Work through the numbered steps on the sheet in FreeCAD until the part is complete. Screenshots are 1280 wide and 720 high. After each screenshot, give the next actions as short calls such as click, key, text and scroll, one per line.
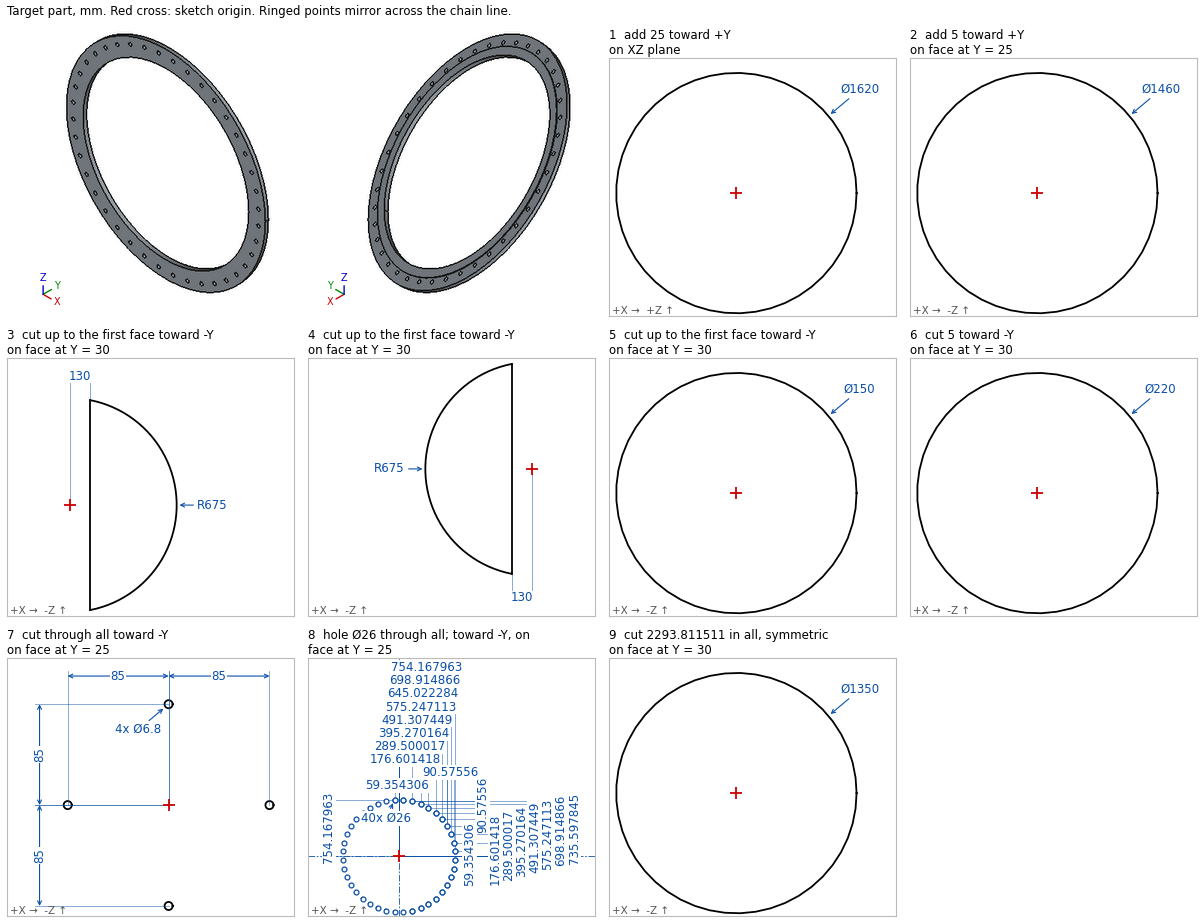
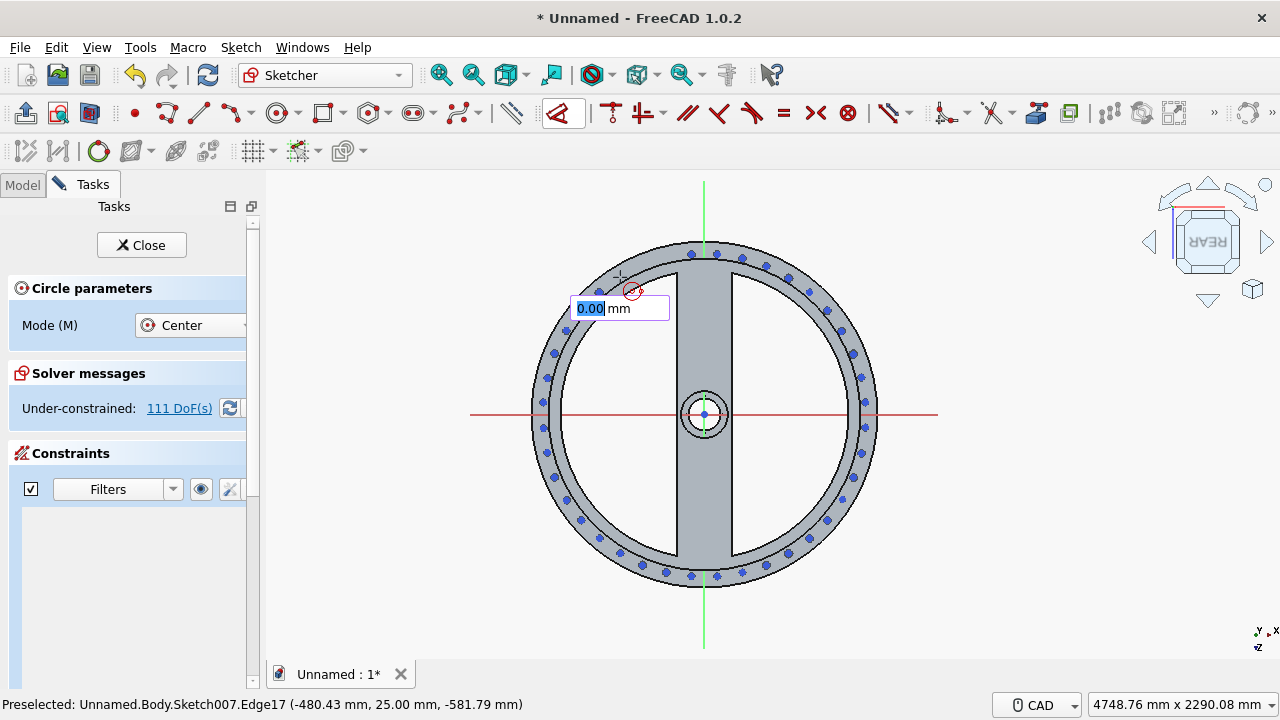
scroll(622, 275, up, 9)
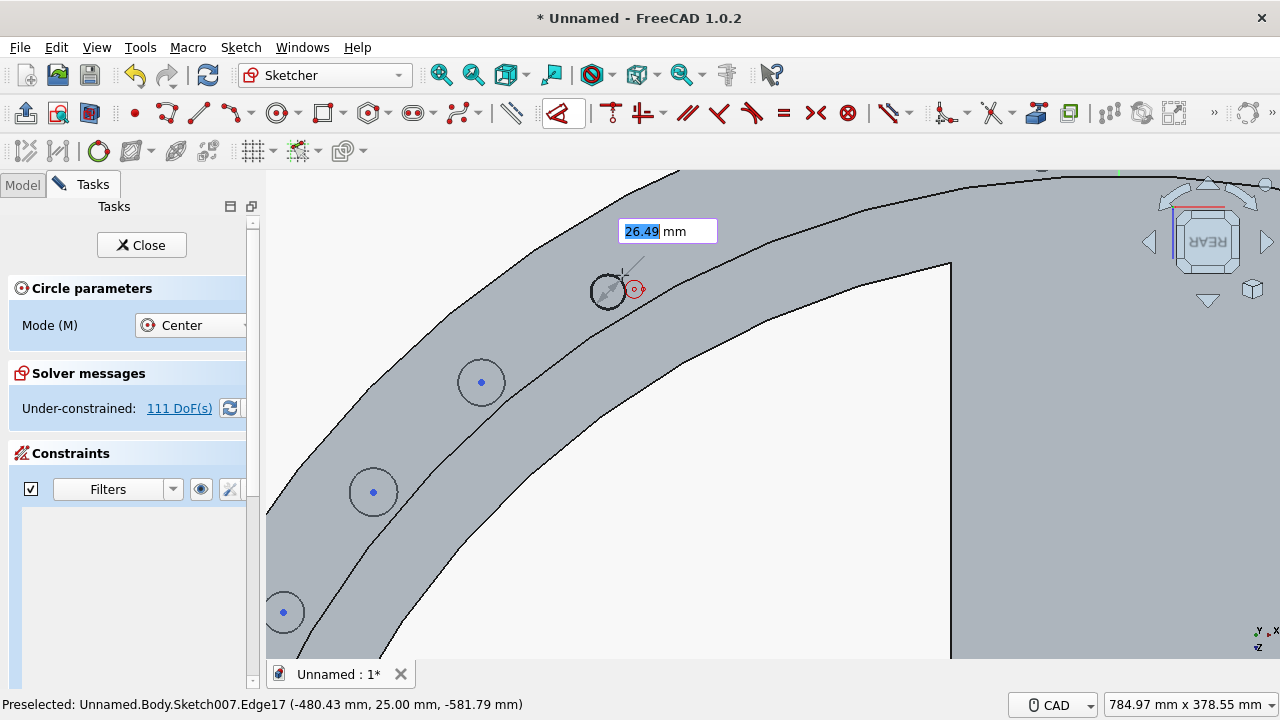
click(620, 273)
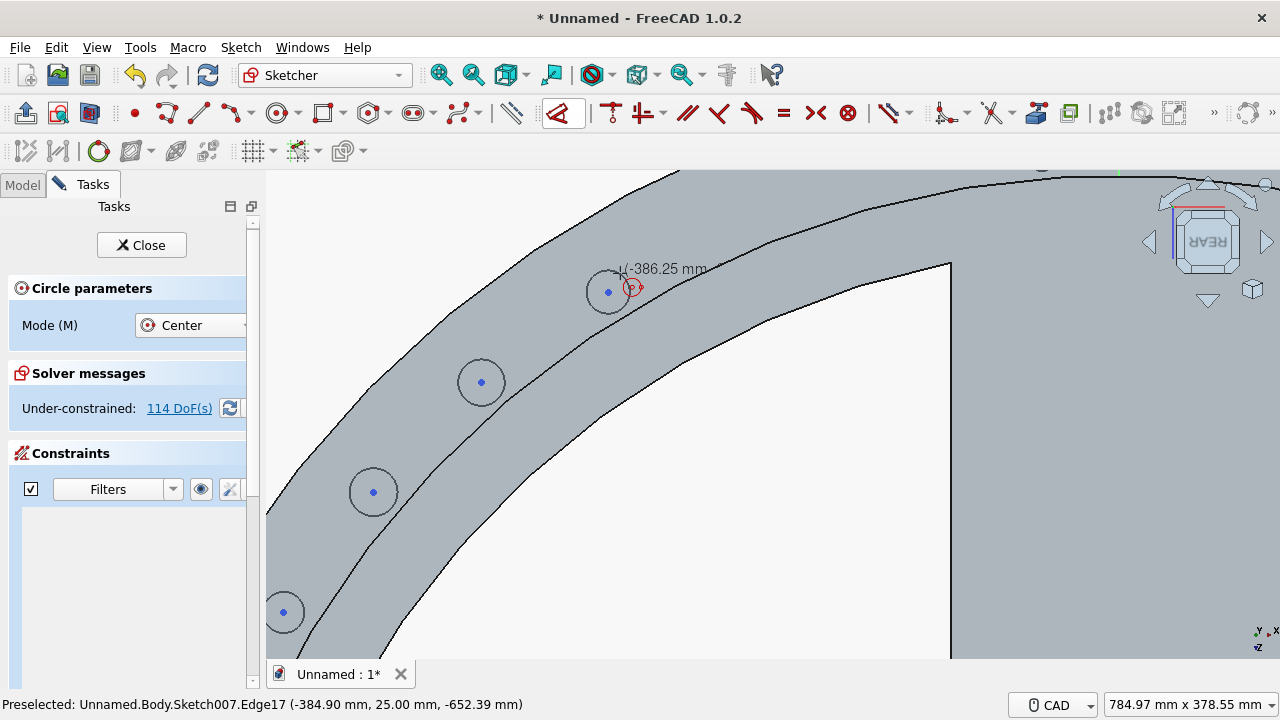
scroll(745, 215, up, 2)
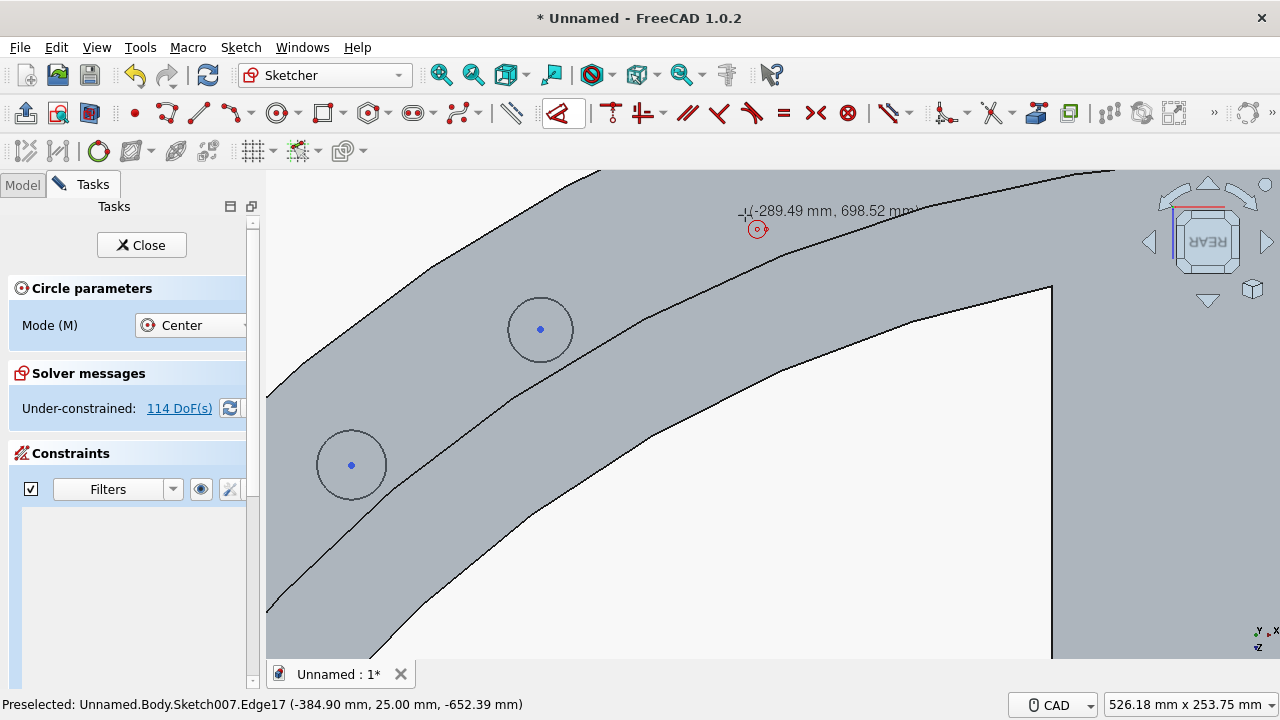
scroll(630, 271, down, 11)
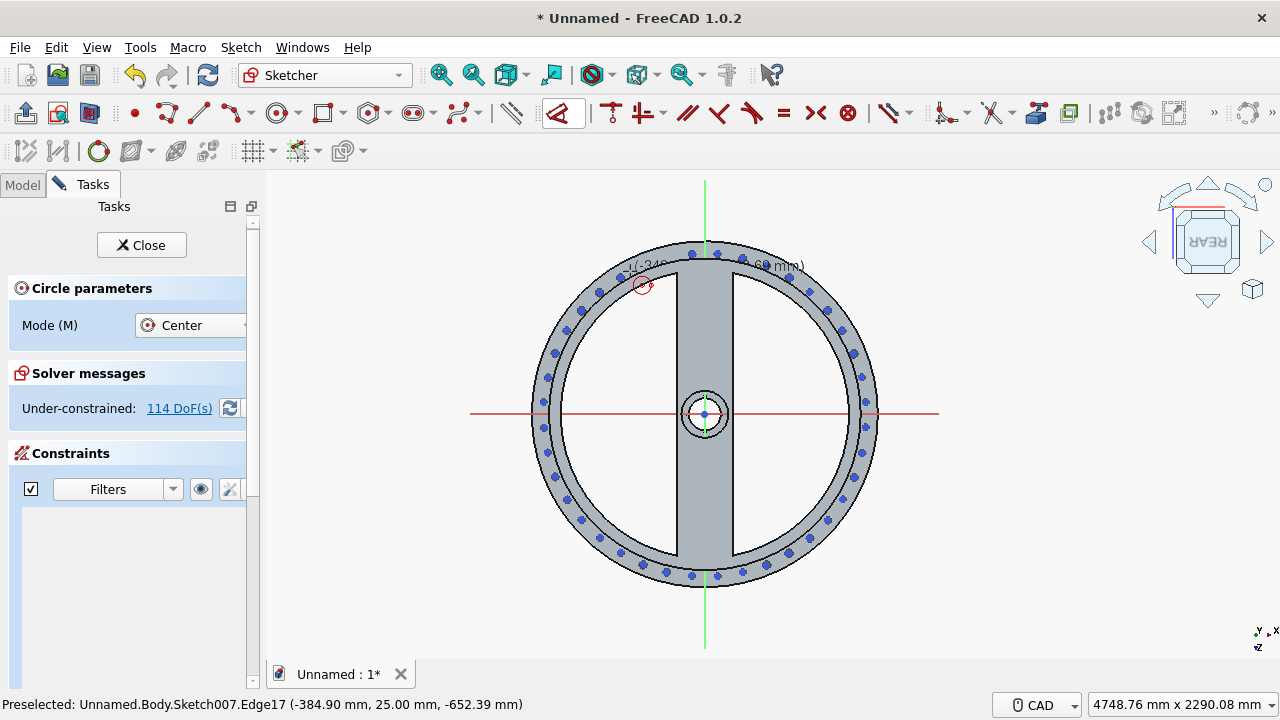
click(643, 265)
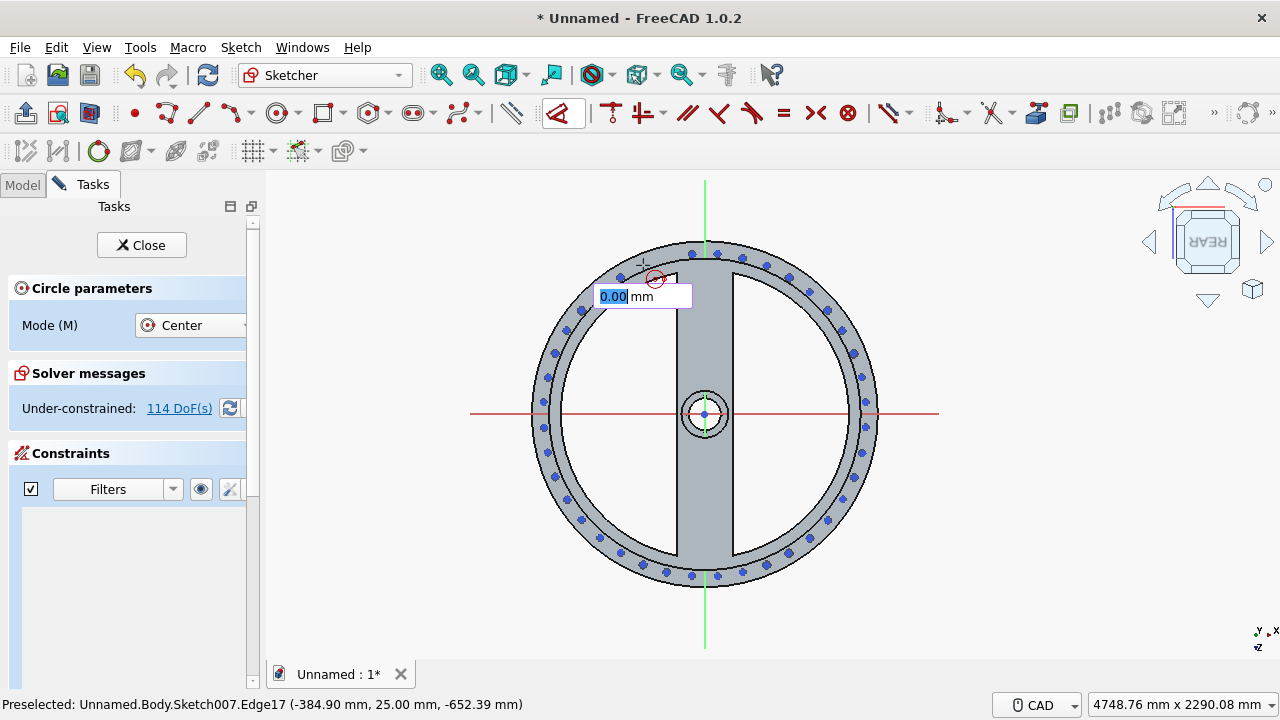
scroll(645, 263, up, 9)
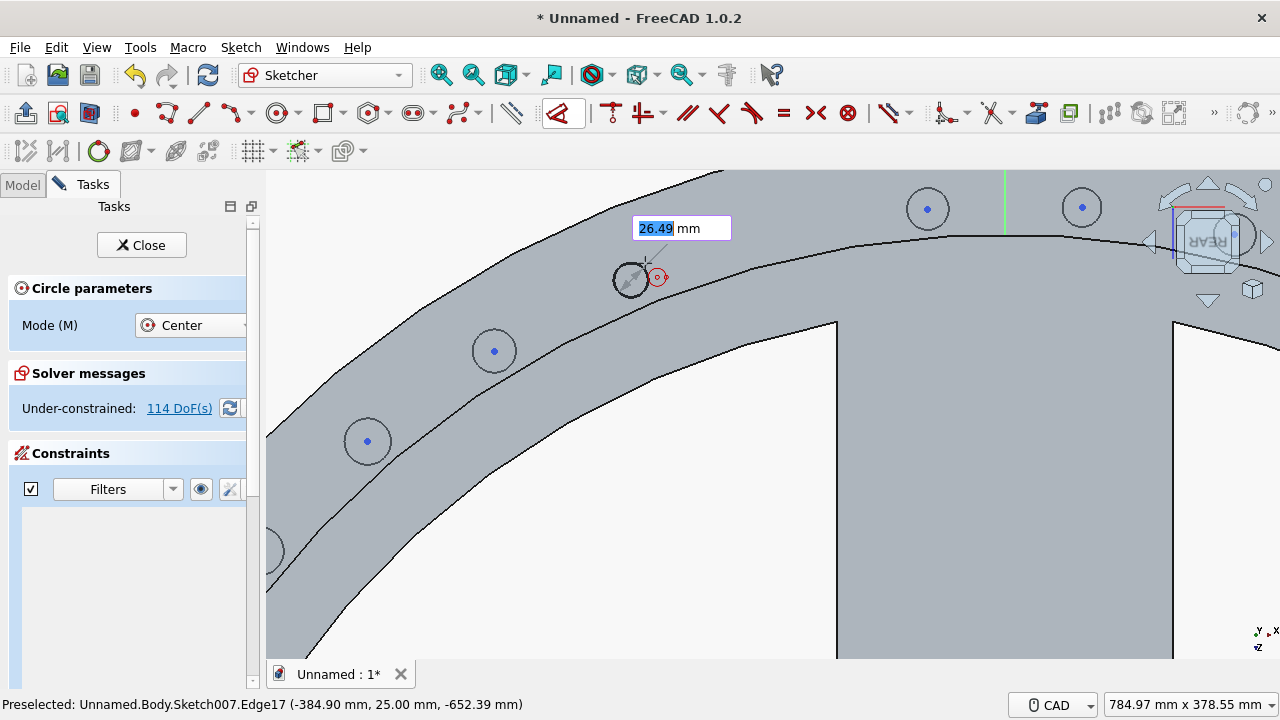
click(643, 263)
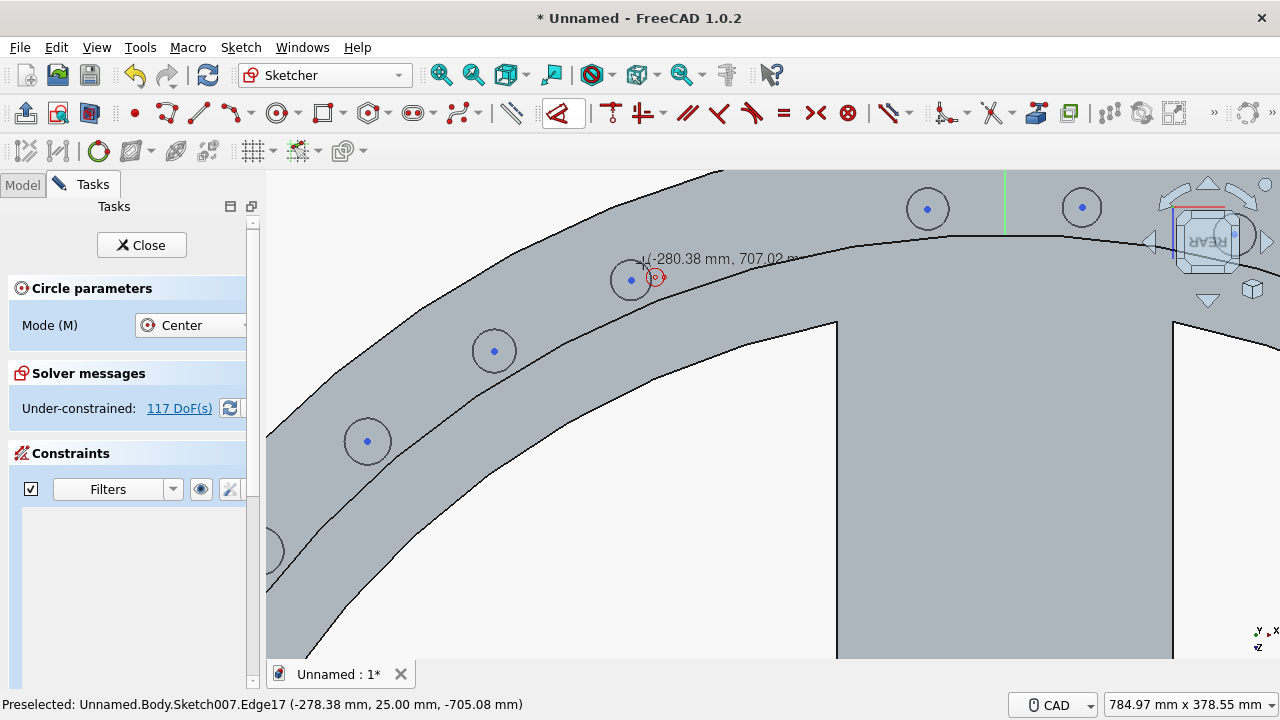
scroll(777, 227, up, 2)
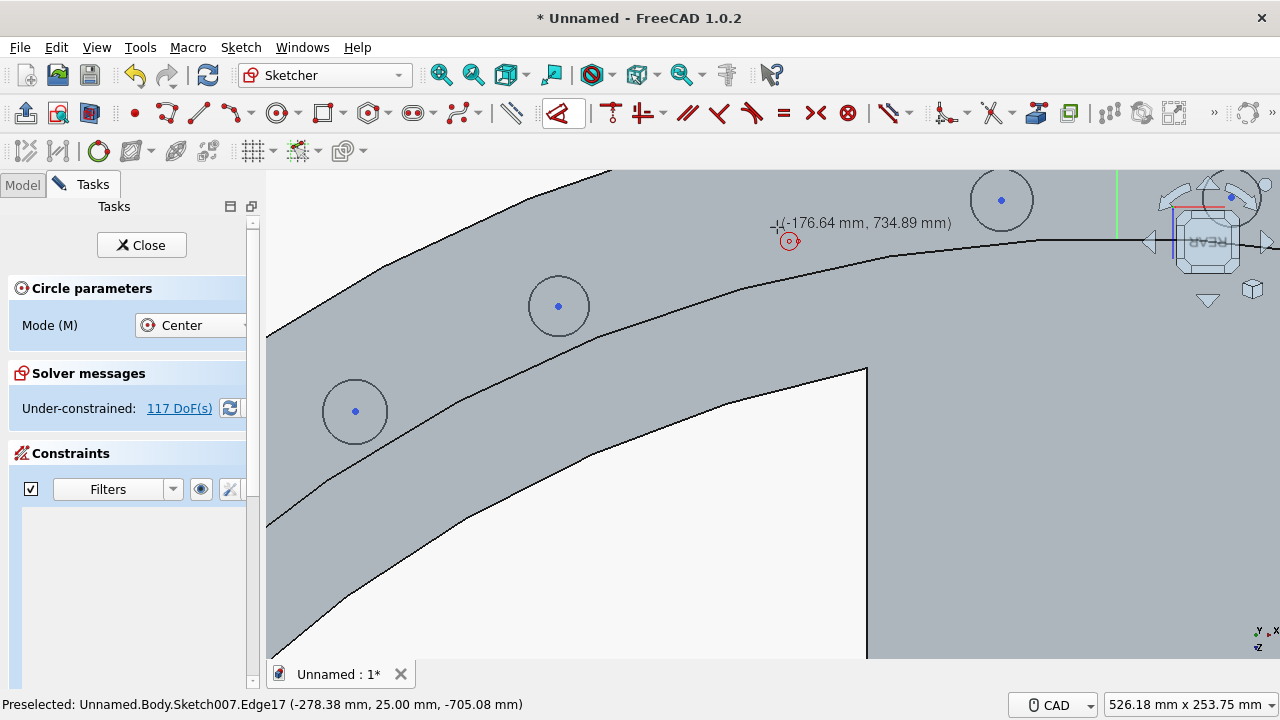
scroll(653, 261, down, 11)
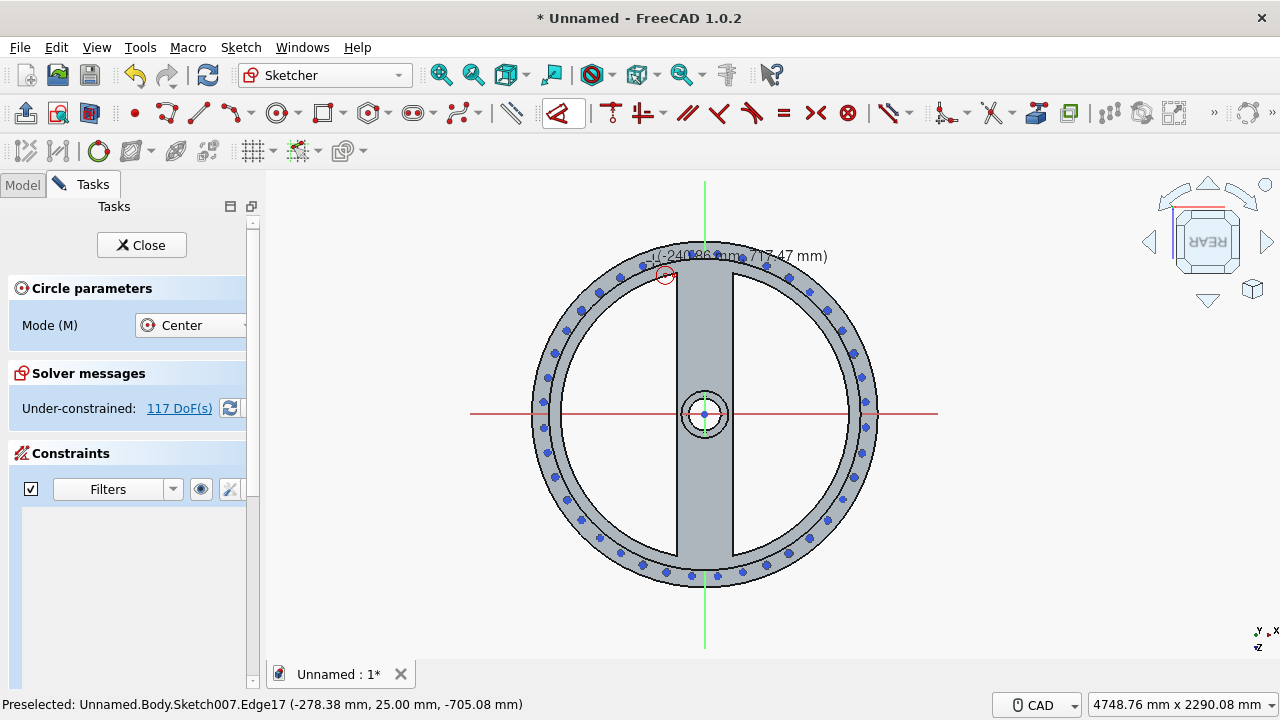
click(667, 257)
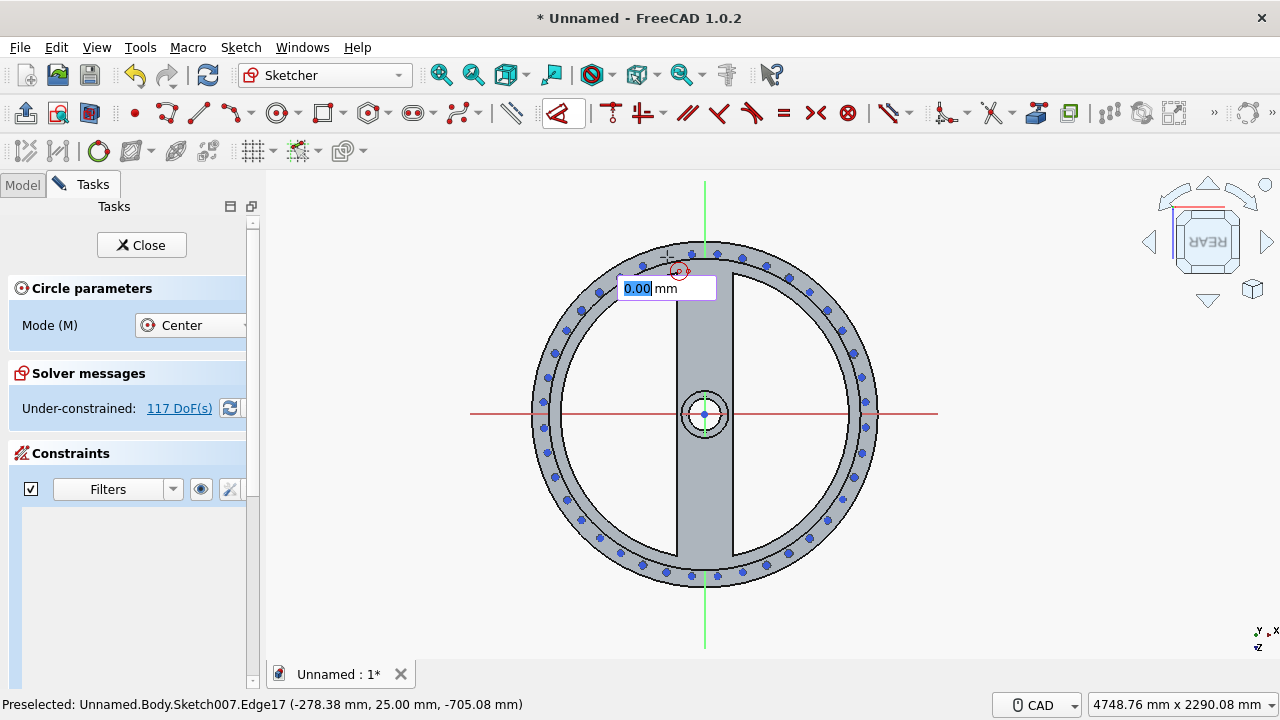
scroll(669, 255, up, 9)